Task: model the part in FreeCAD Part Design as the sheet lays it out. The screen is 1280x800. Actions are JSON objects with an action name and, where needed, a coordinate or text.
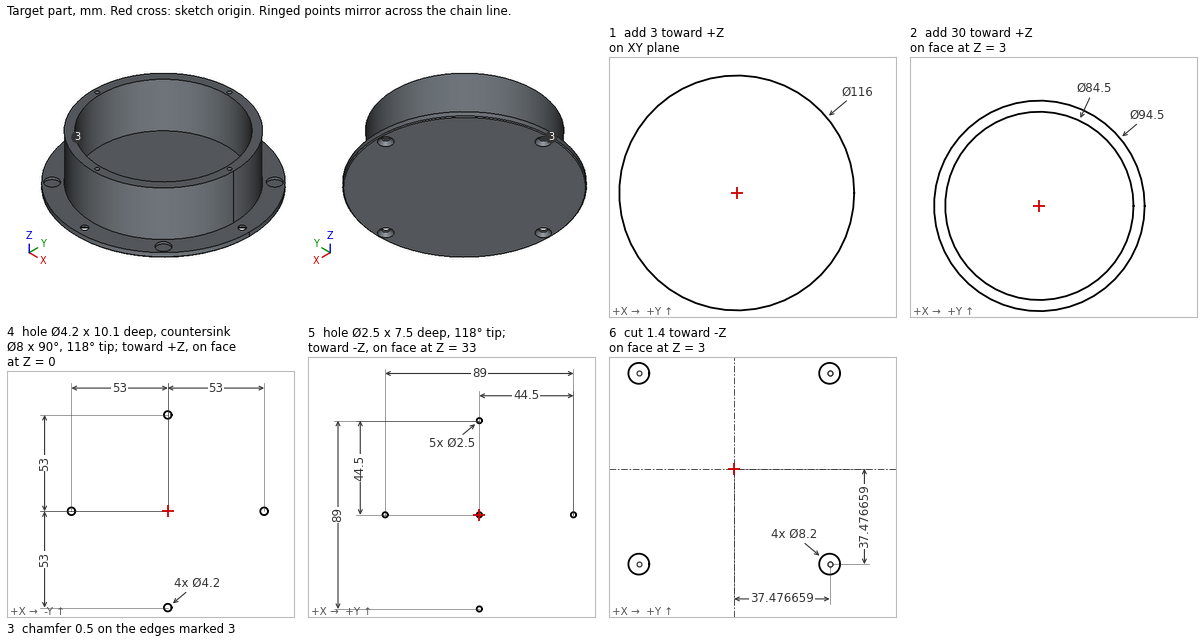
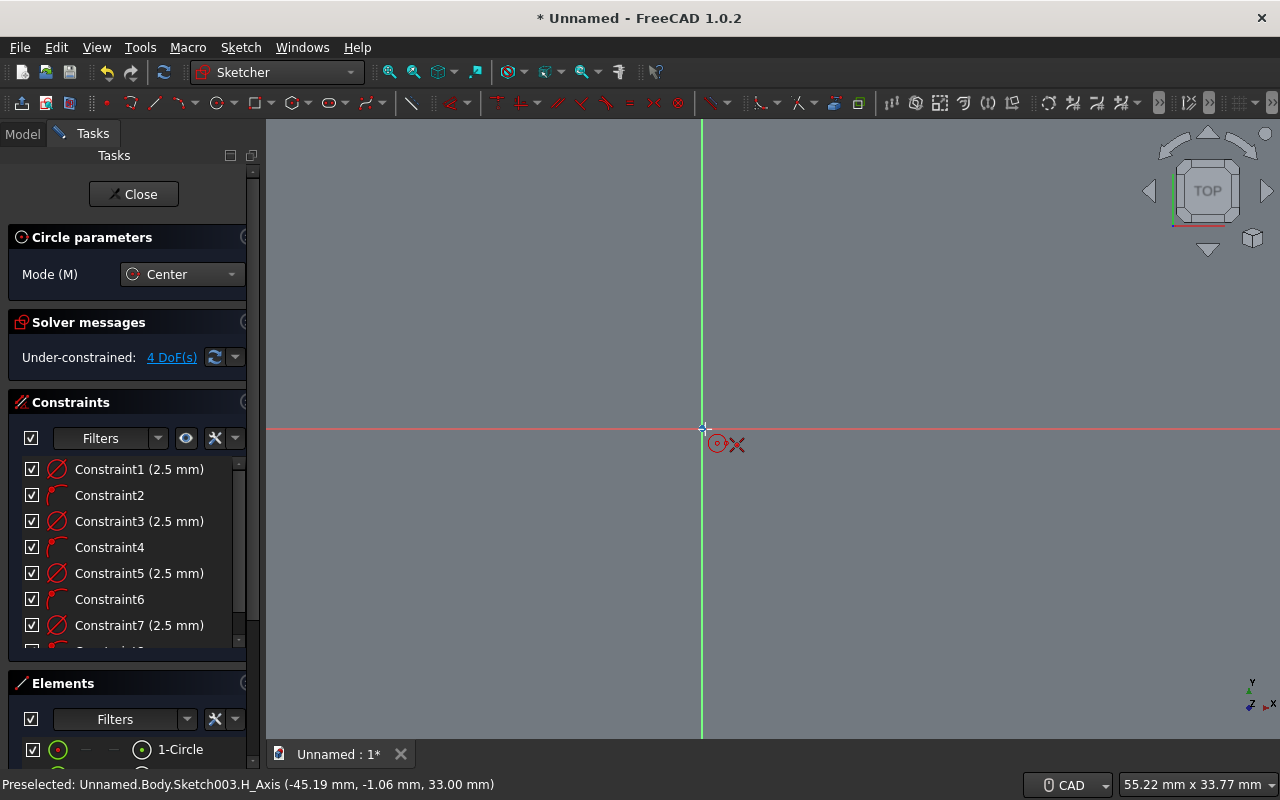
{"action": "scroll", "coordinate": [705, 429], "scroll_direction": "down", "scroll_amount": 7}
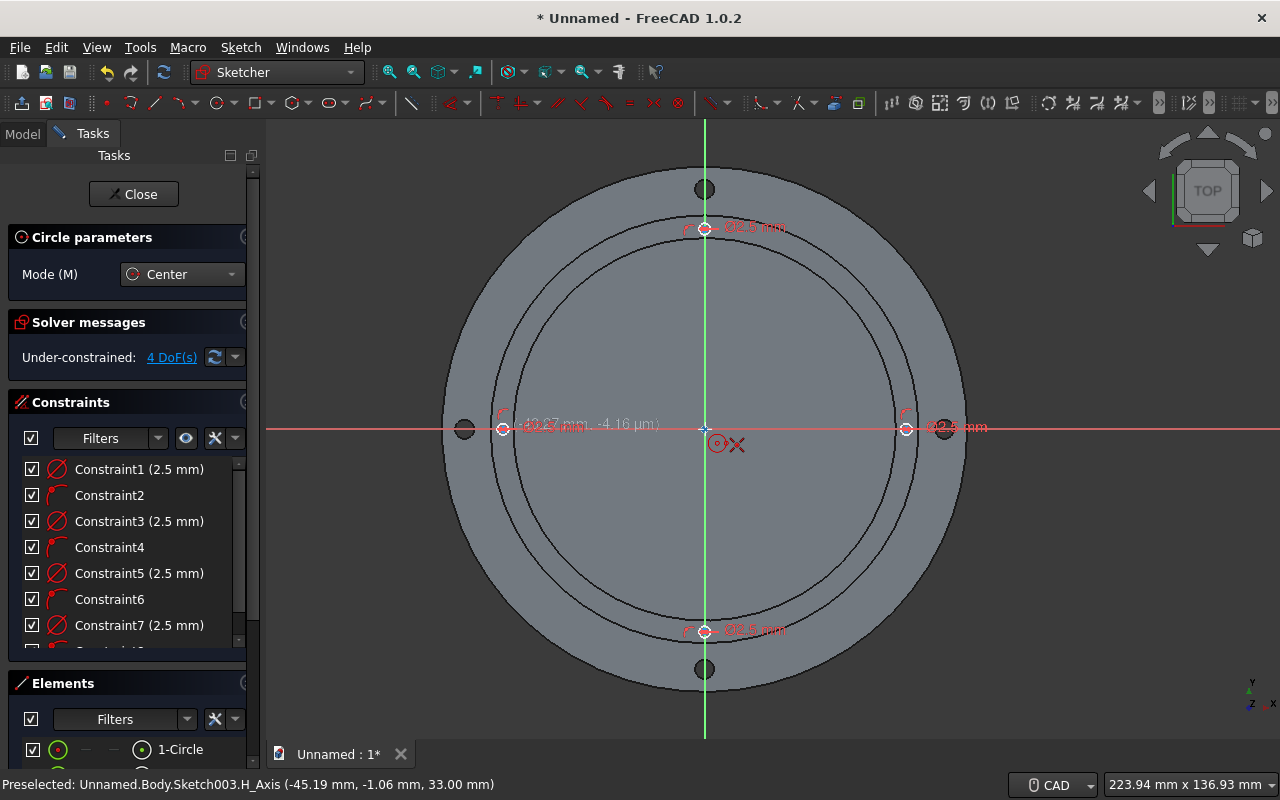
{"action": "left_click", "coordinate": [705, 429]}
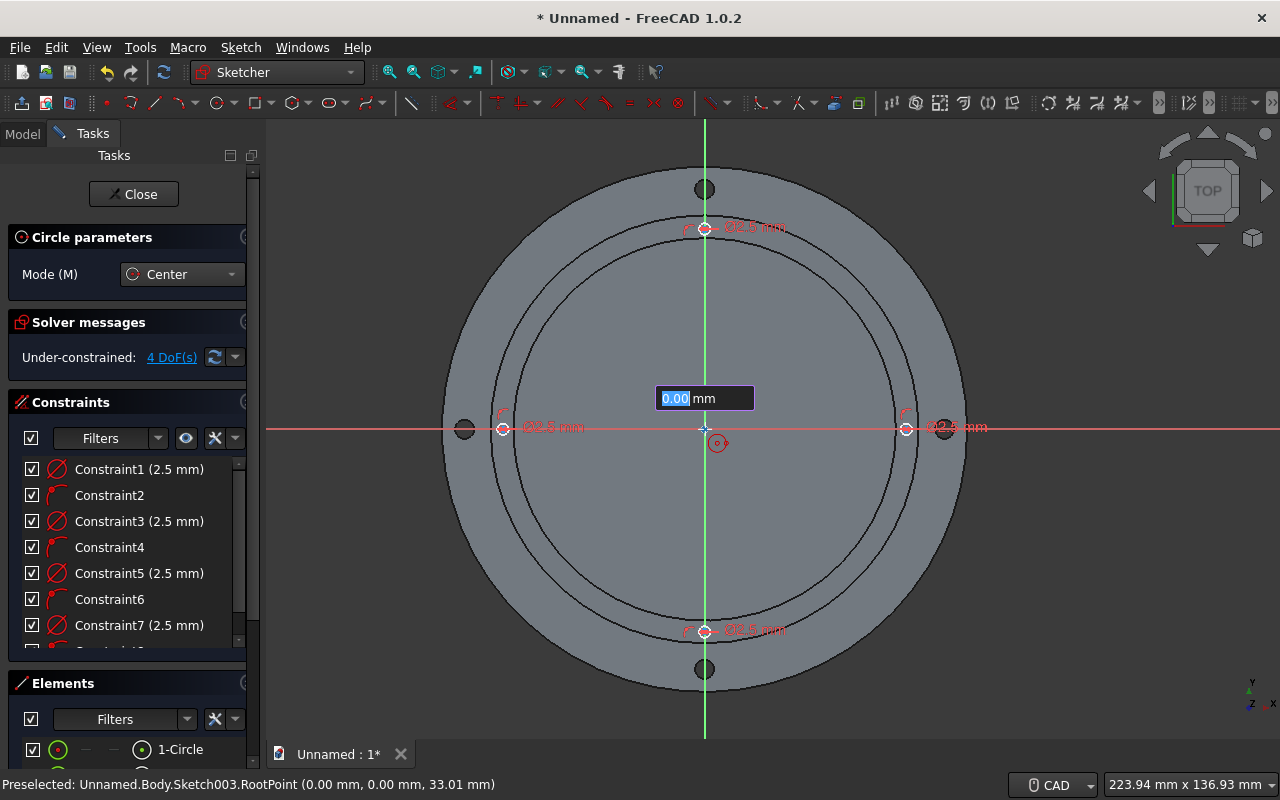
{"action": "scroll", "coordinate": [709, 425], "scroll_direction": "up", "scroll_amount": 7}
{"action": "mouse_move", "coordinate": [706, 425]}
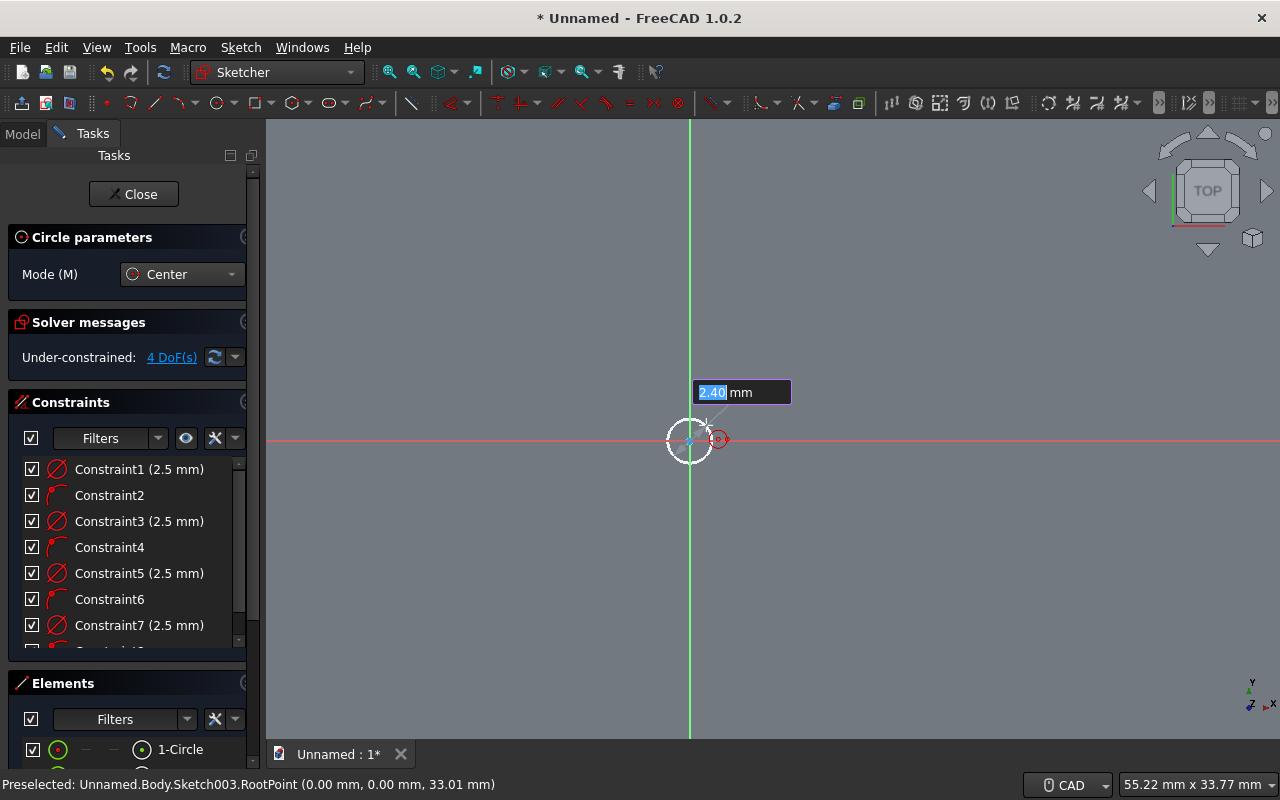
{"action": "type", "text": "2.5"}
{"action": "key", "text": "Return"}
{"action": "key", "text": "Escape"}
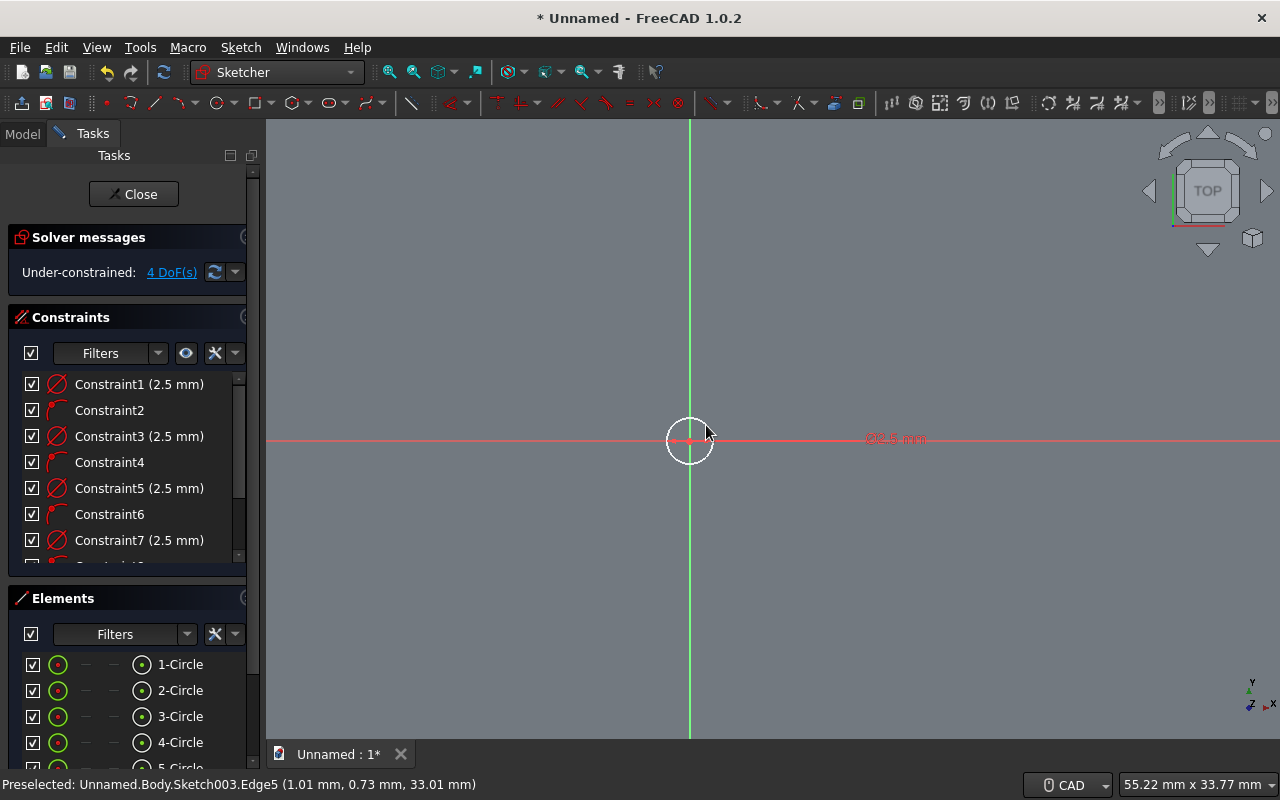
{"action": "left_click", "coordinate": [450, 104]}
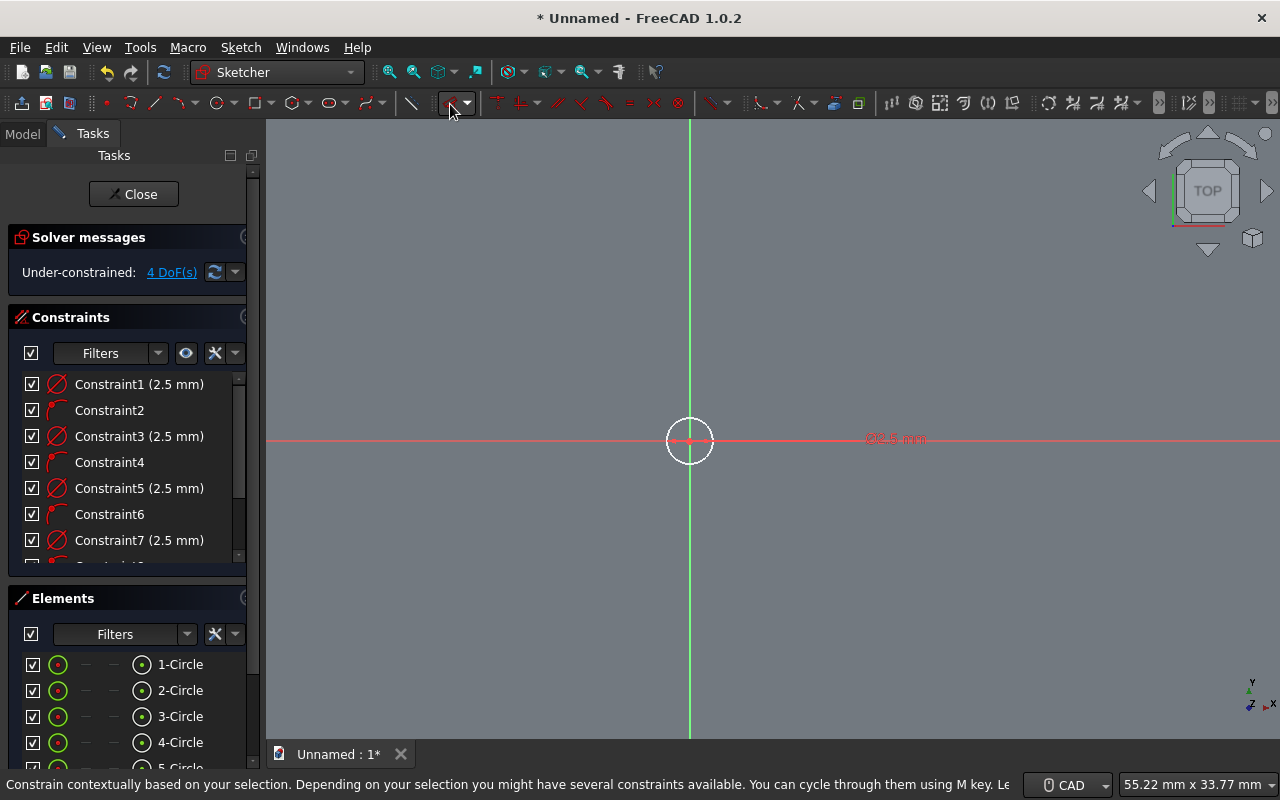
{"action": "scroll", "coordinate": [709, 425], "scroll_direction": "down", "scroll_amount": 7}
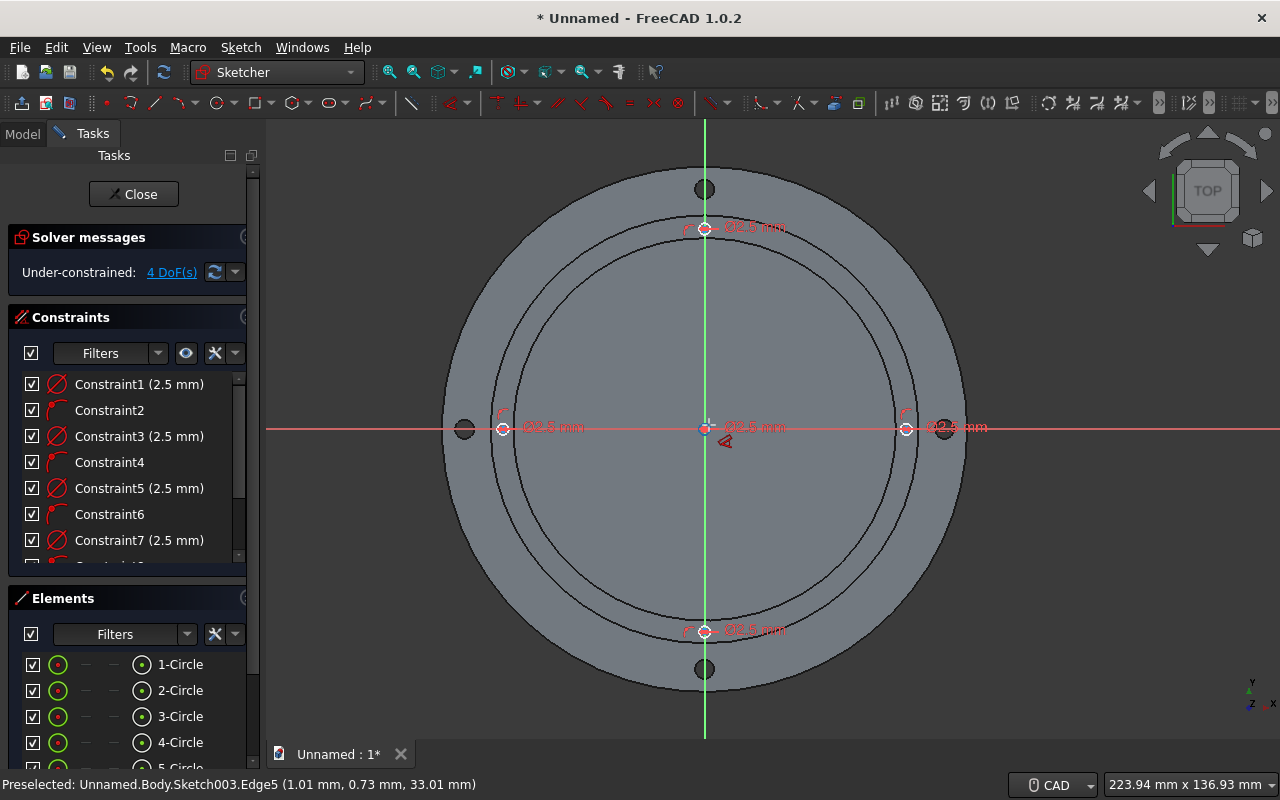
{"action": "left_click", "coordinate": [705, 229]}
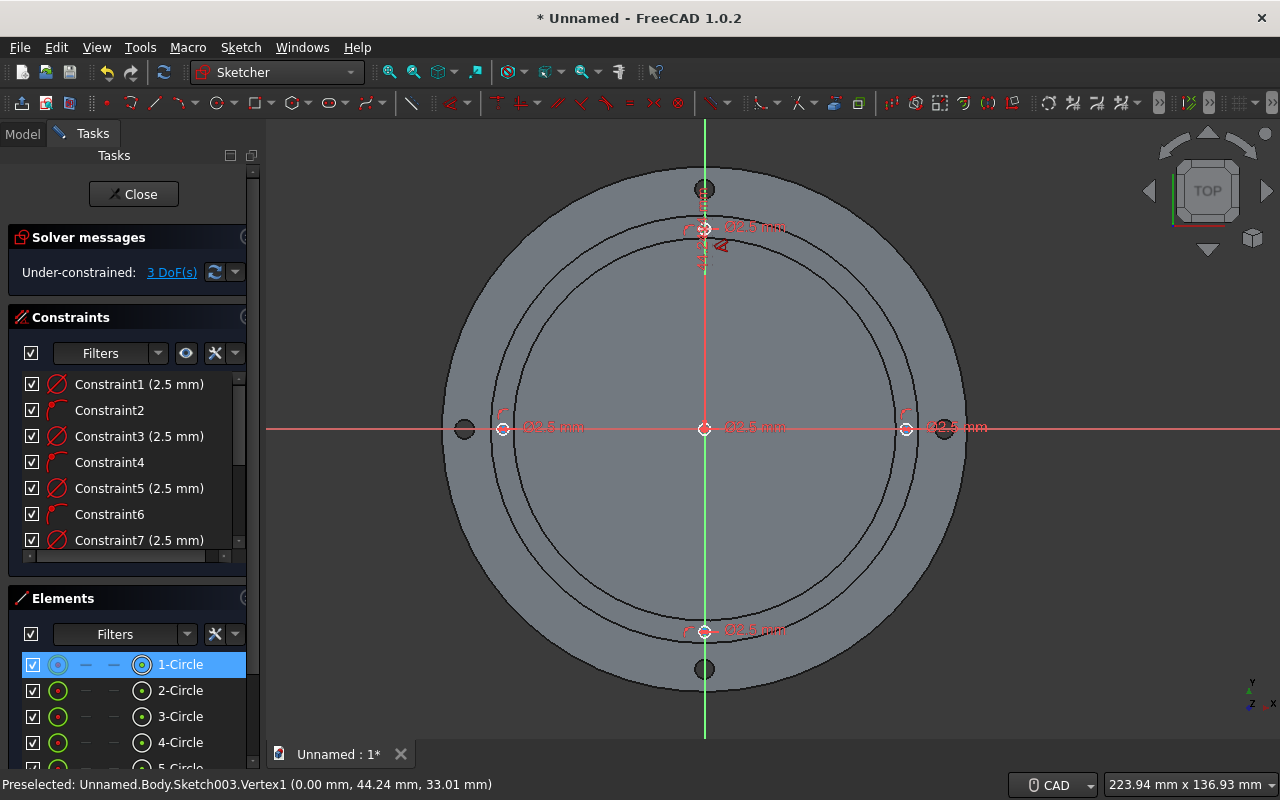
{"action": "left_click", "coordinate": [705, 632]}
{"action": "left_click", "coordinate": [739, 338]}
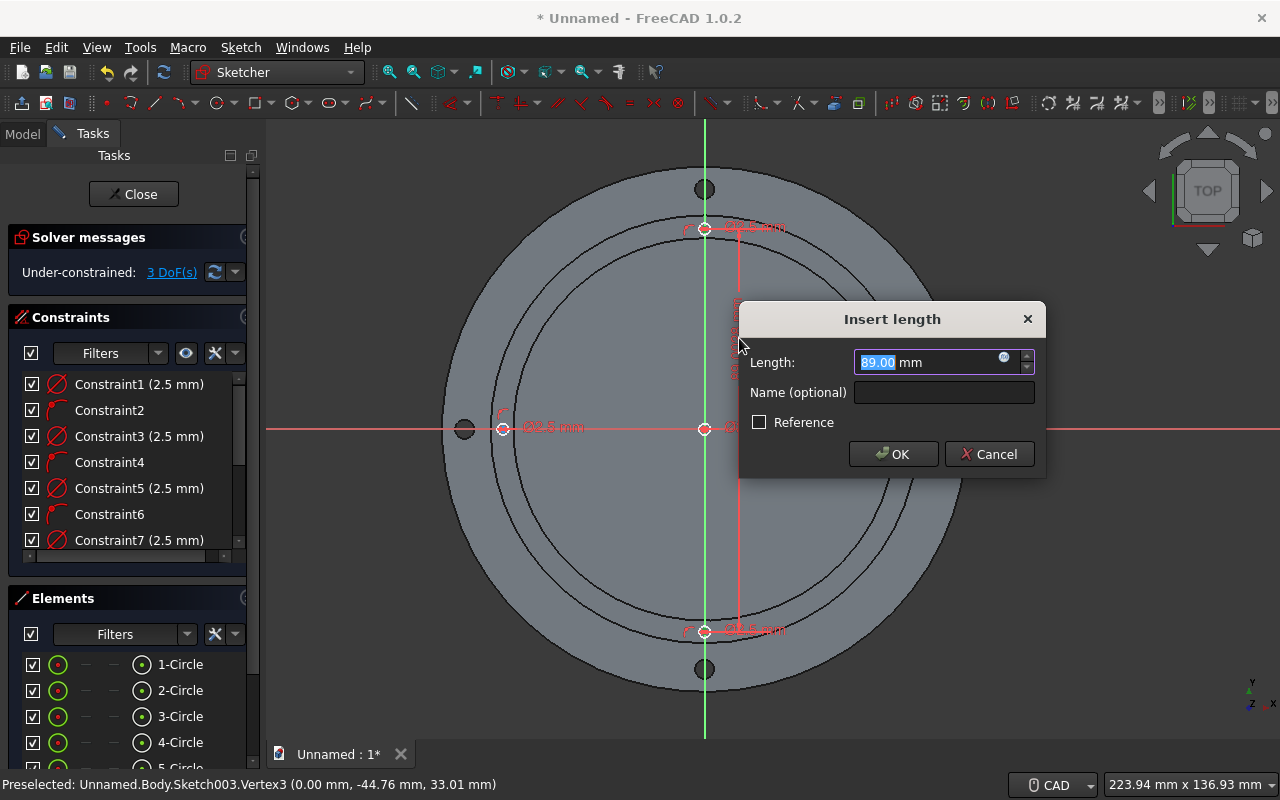
{"action": "type", "text": "89"}
{"action": "key", "text": "Return"}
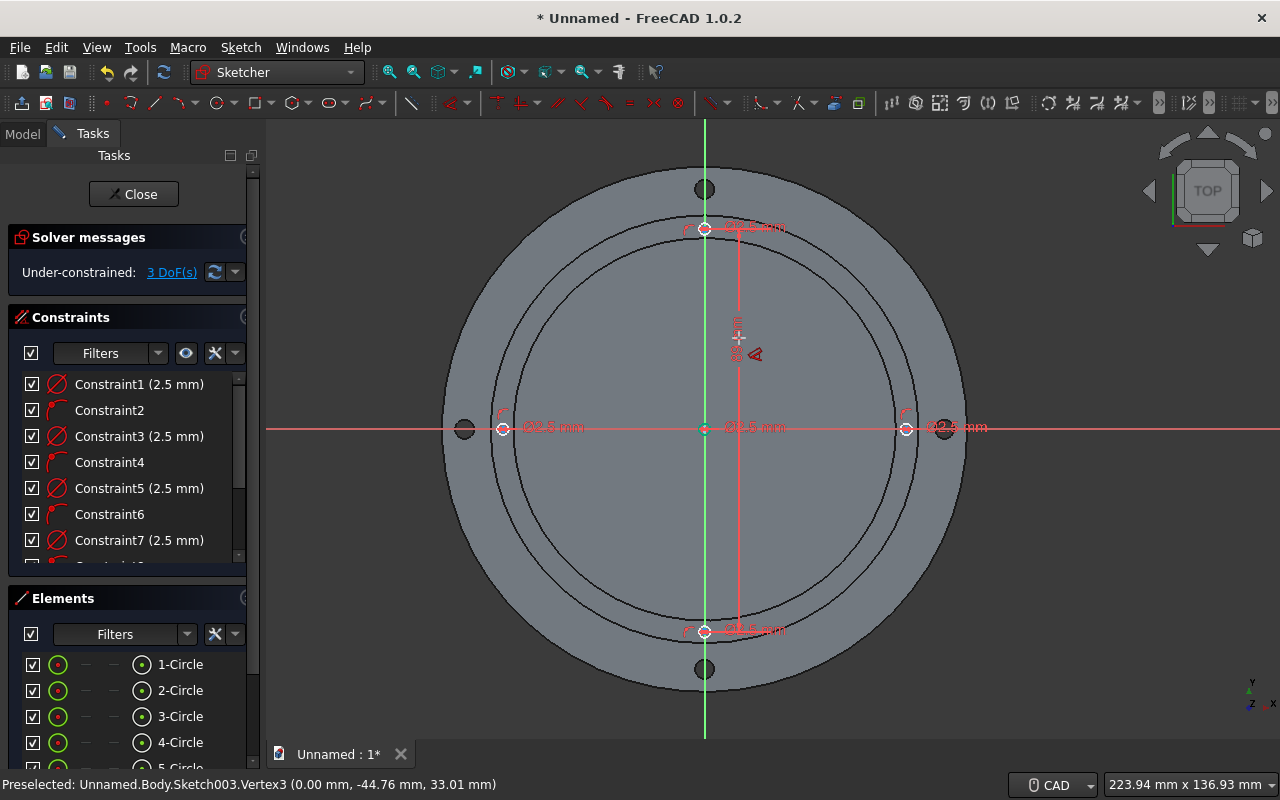
{"action": "left_click", "coordinate": [906, 429]}